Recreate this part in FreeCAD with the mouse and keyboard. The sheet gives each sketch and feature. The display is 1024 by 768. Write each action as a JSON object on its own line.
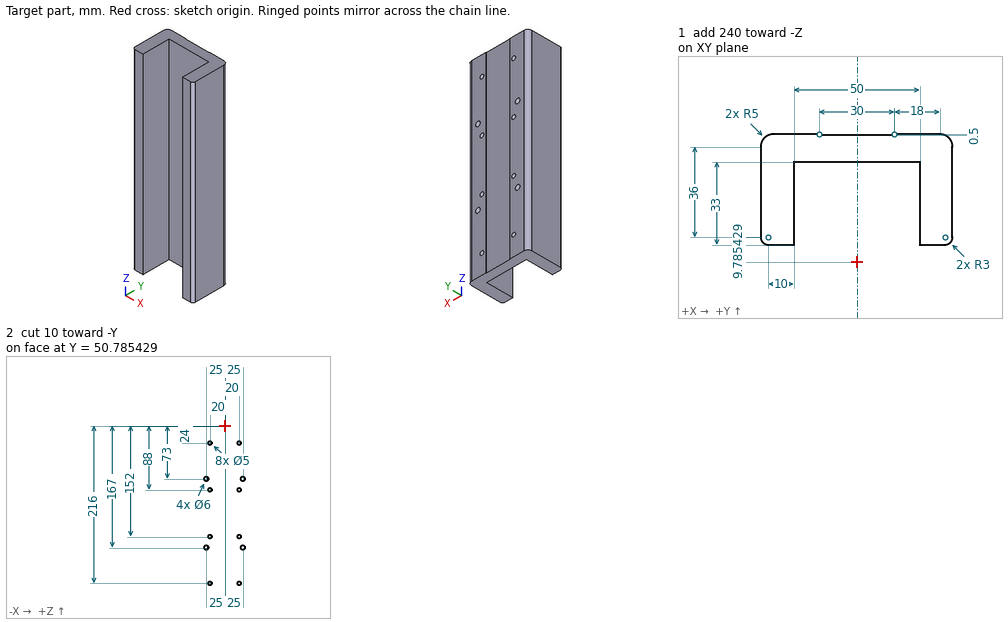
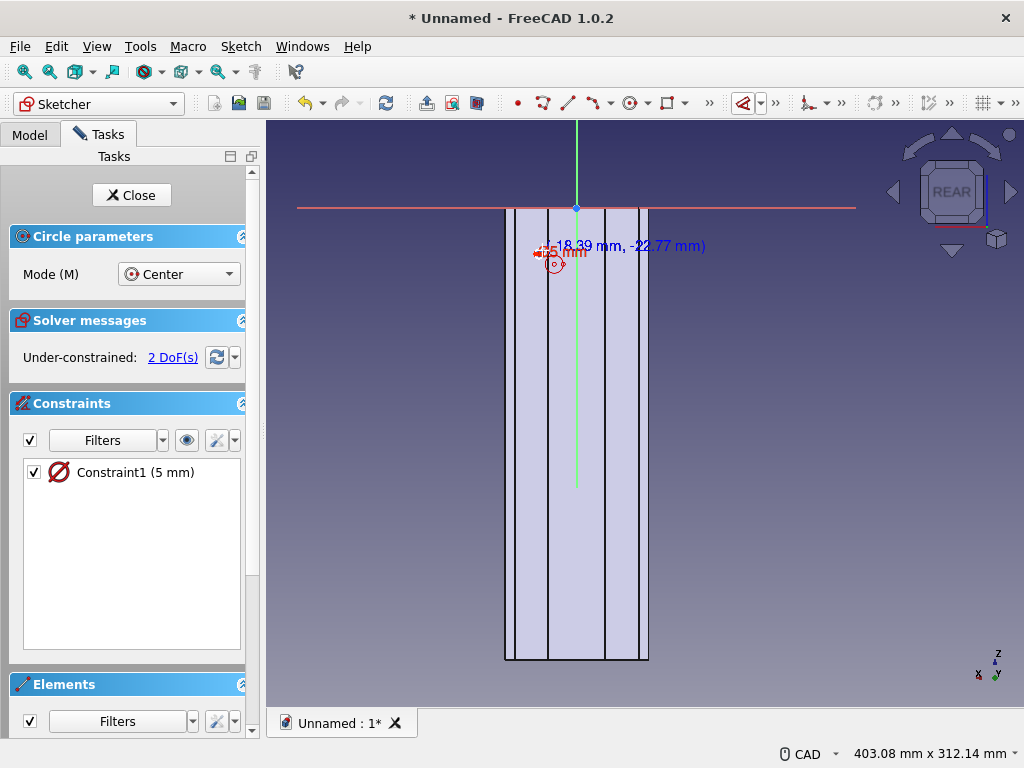
{"action": "scroll", "coordinate": [614, 253], "scroll_direction": "up", "scroll_amount": 8}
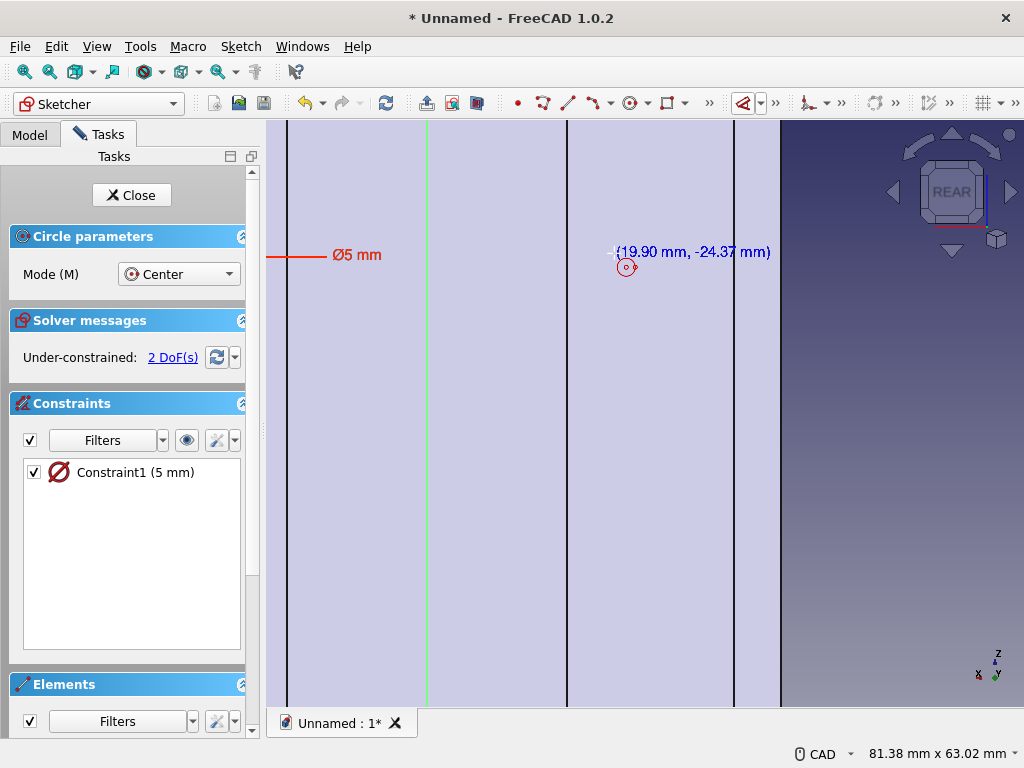
{"action": "scroll", "coordinate": [614, 253], "scroll_direction": "down", "scroll_amount": 8}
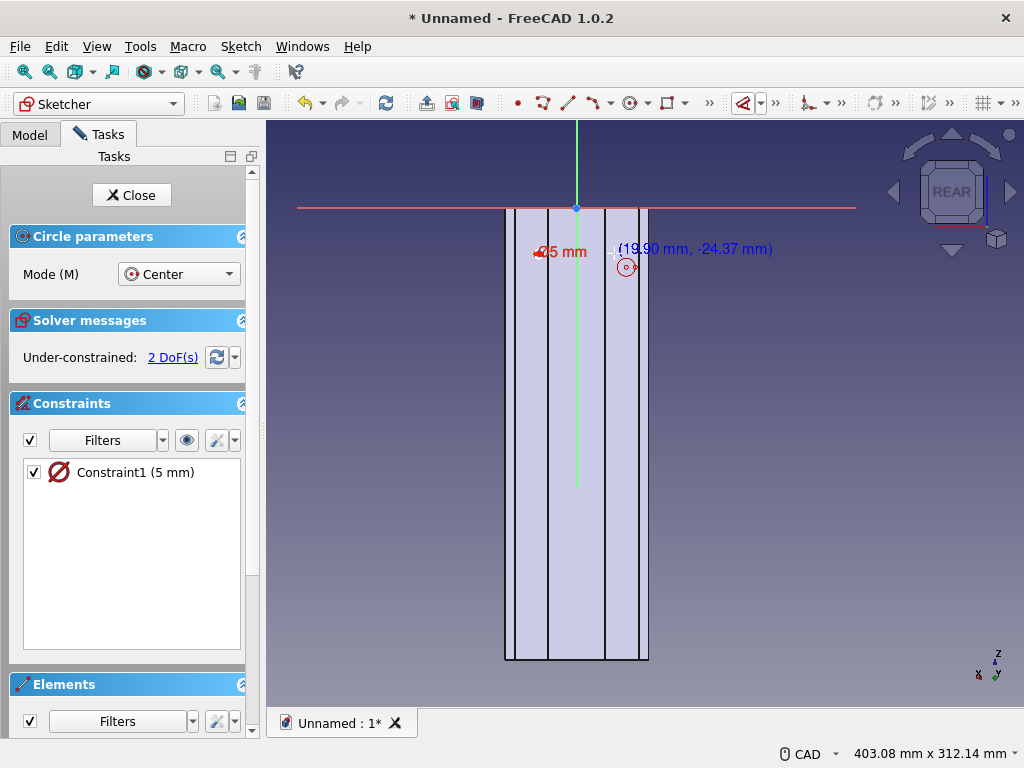
{"action": "left_click", "coordinate": [614, 253]}
{"action": "mouse_move", "coordinate": [618, 250]}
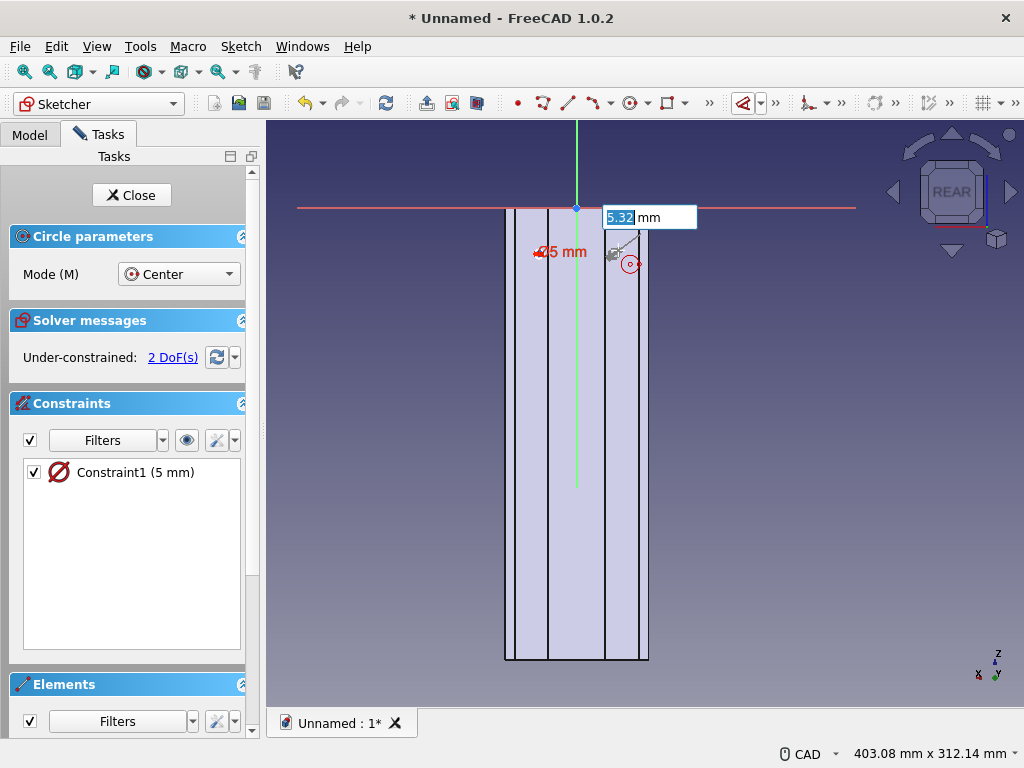
{"action": "type", "text": "5"}
{"action": "key", "text": "Return"}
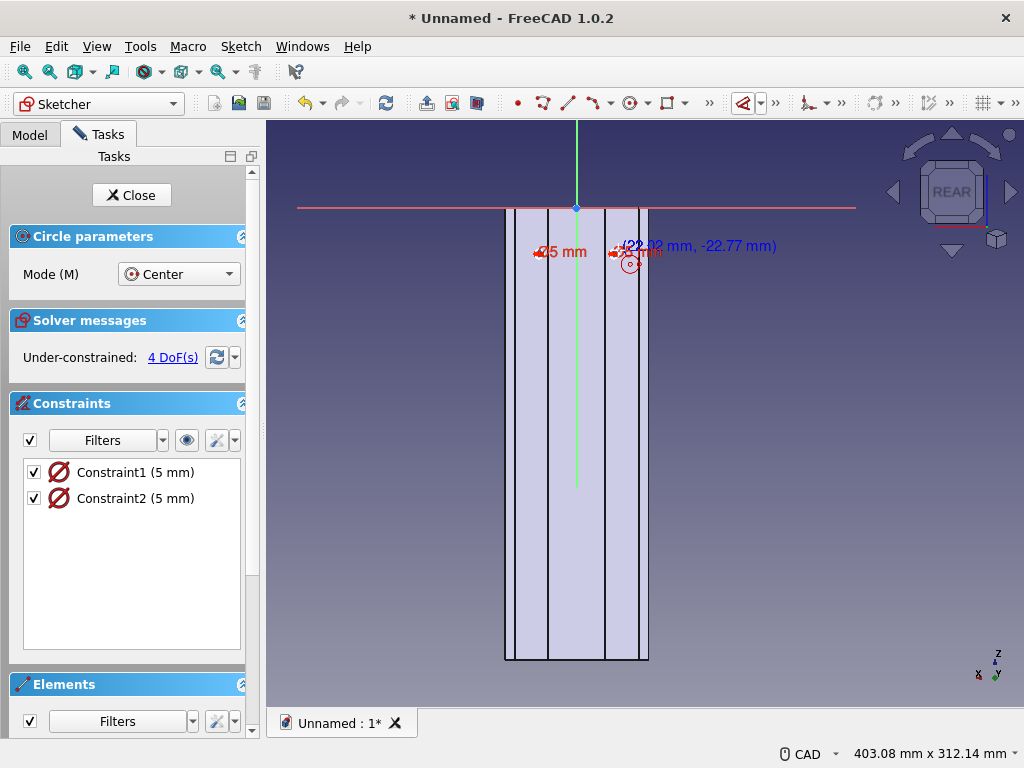
{"action": "scroll", "coordinate": [539, 374], "scroll_direction": "up", "scroll_amount": 8}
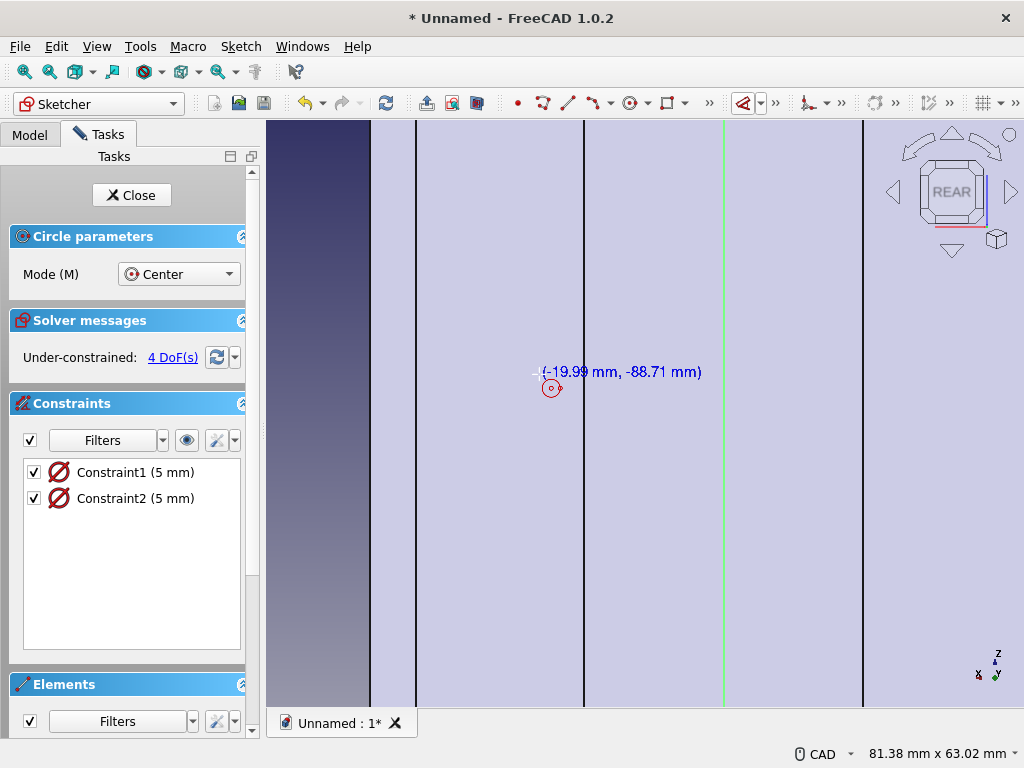
{"action": "scroll", "coordinate": [539, 374], "scroll_direction": "down", "scroll_amount": 8}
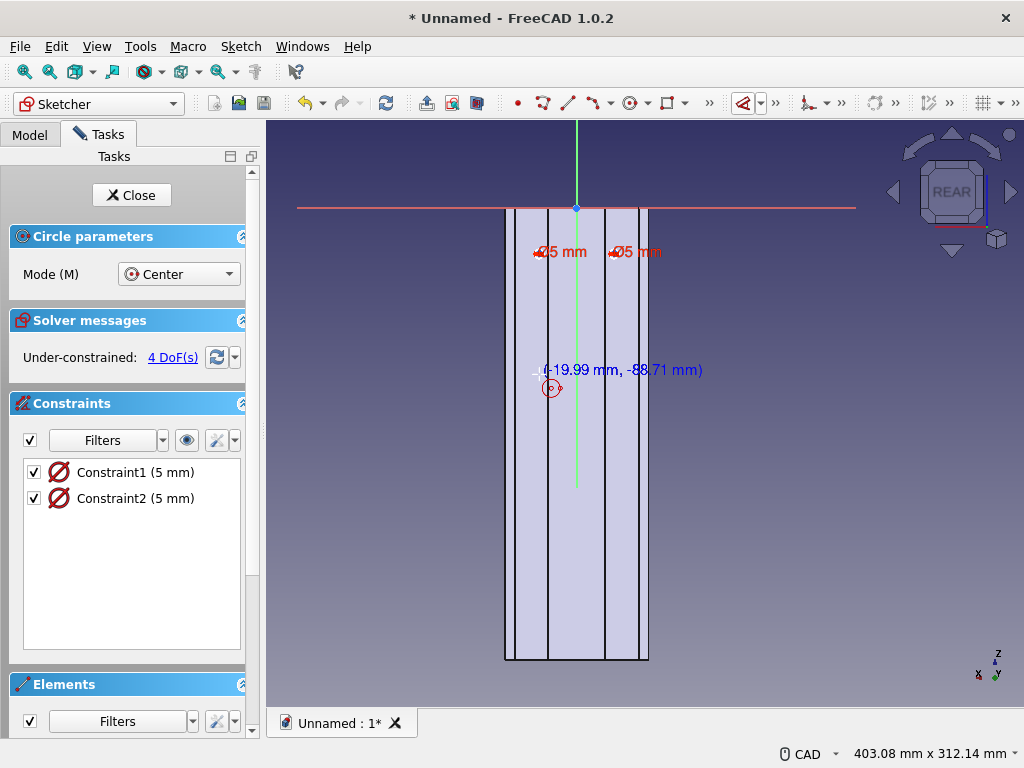
{"action": "left_click", "coordinate": [539, 374]}
{"action": "mouse_move", "coordinate": [542, 370]}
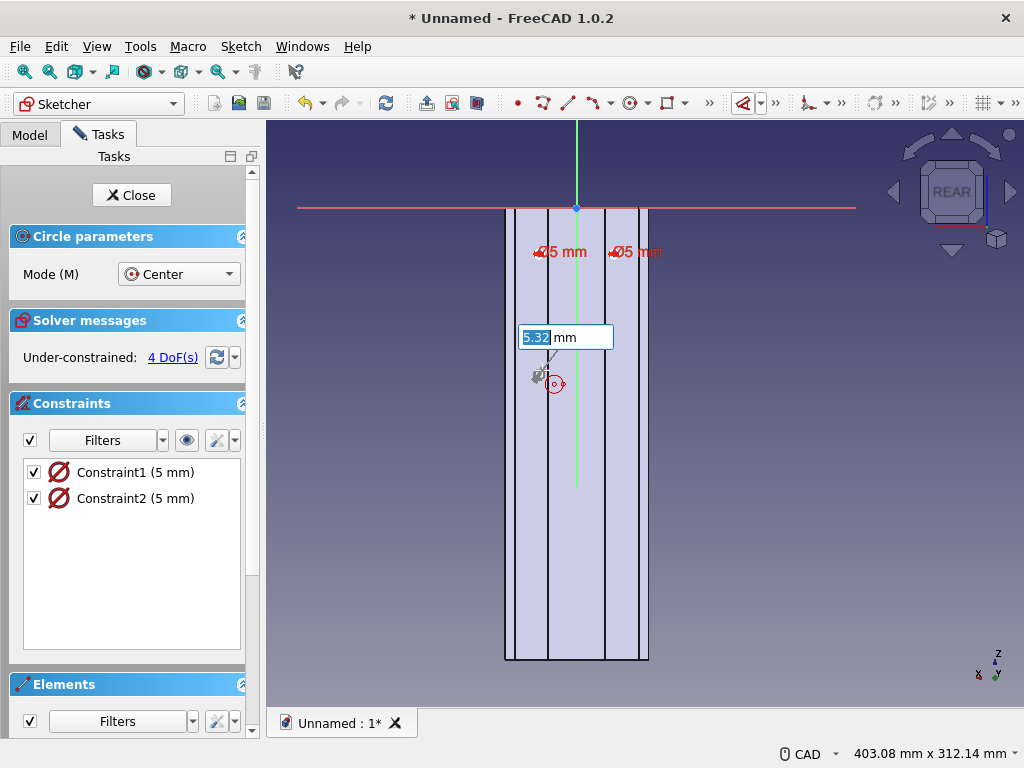
{"action": "type", "text": "5"}
{"action": "key", "text": "Return"}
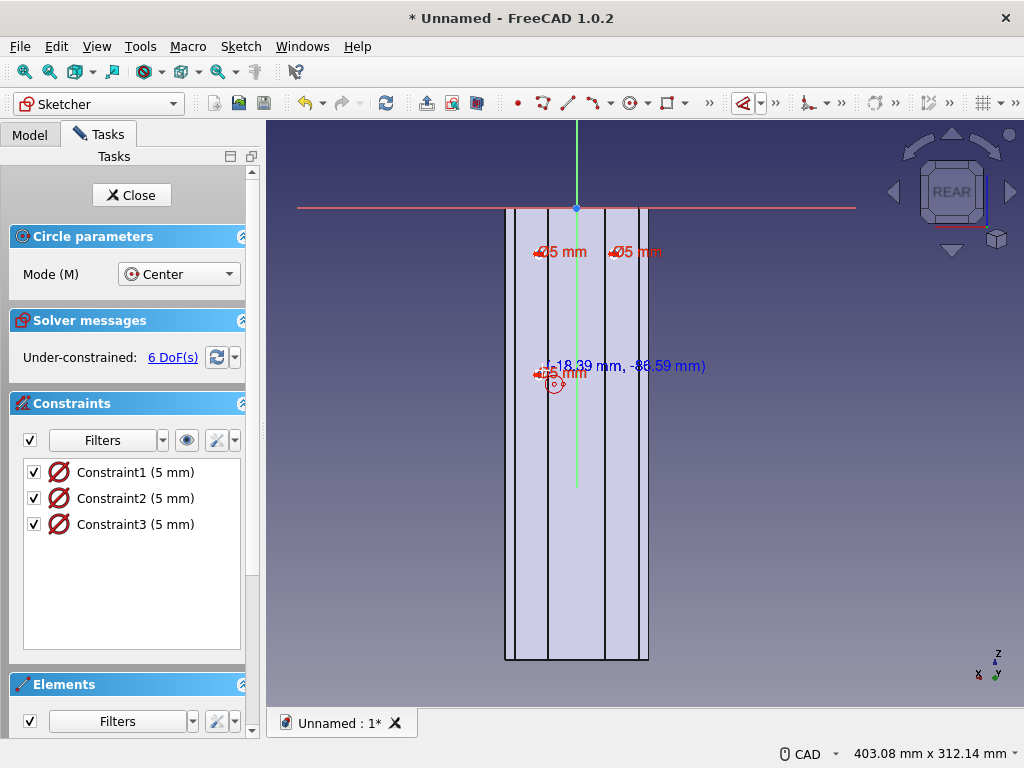
{"action": "scroll", "coordinate": [614, 374], "scroll_direction": "up", "scroll_amount": 8}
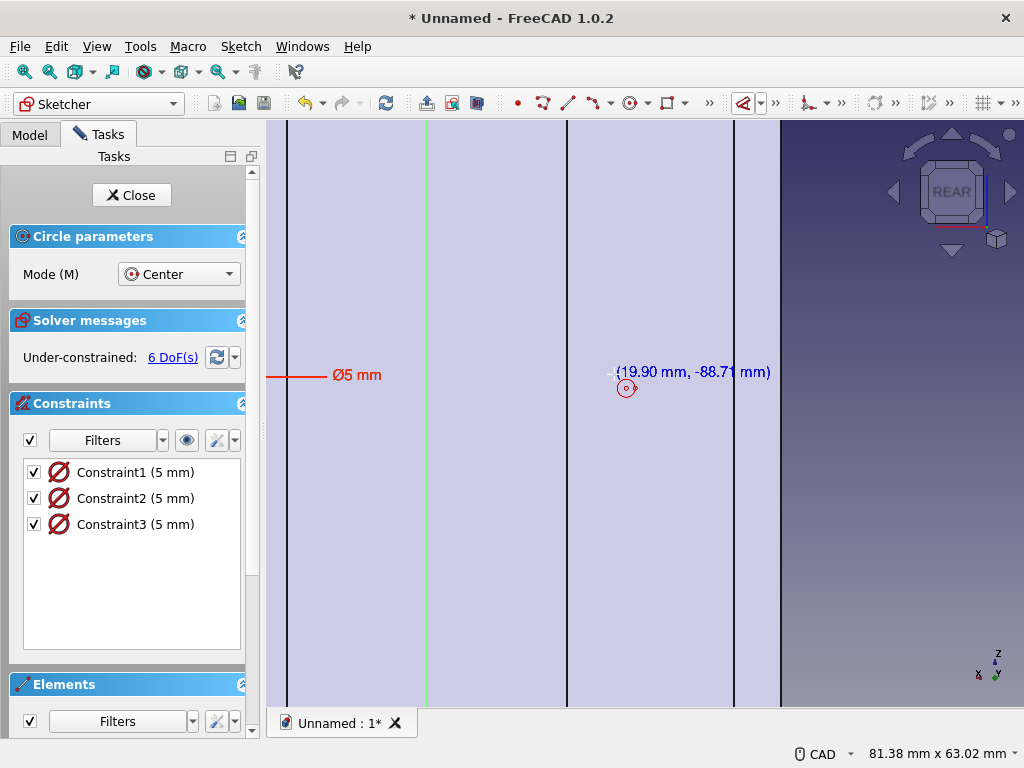
{"action": "scroll", "coordinate": [614, 374], "scroll_direction": "down", "scroll_amount": 8}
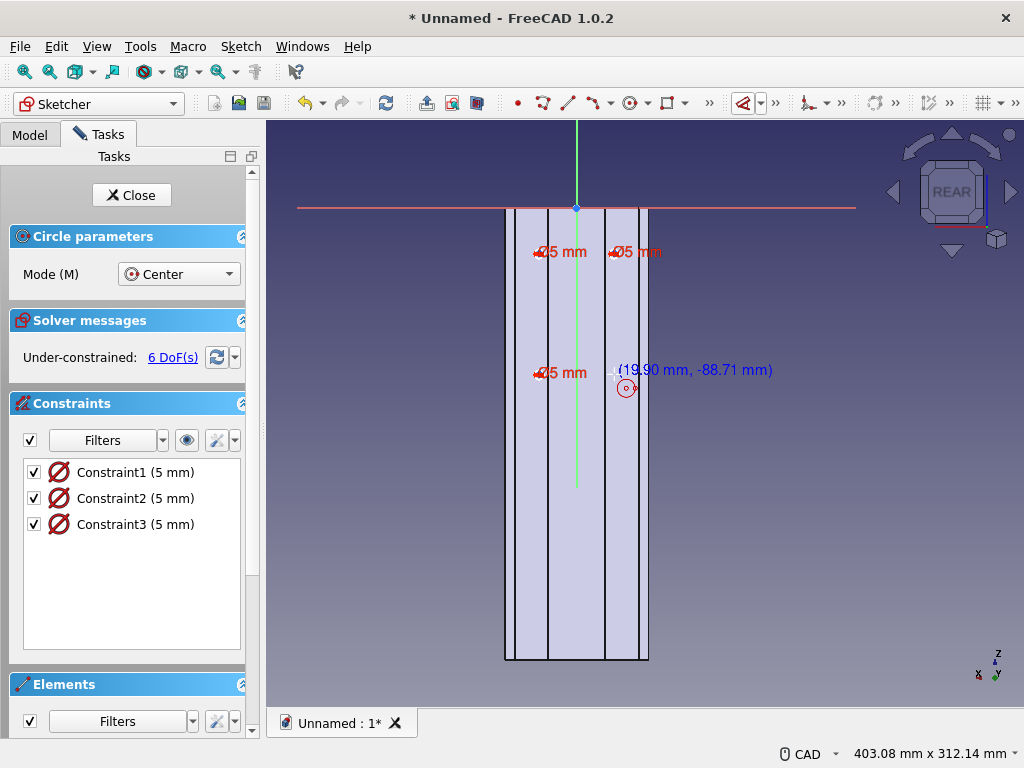
{"action": "left_click", "coordinate": [614, 374]}
{"action": "mouse_move", "coordinate": [618, 370]}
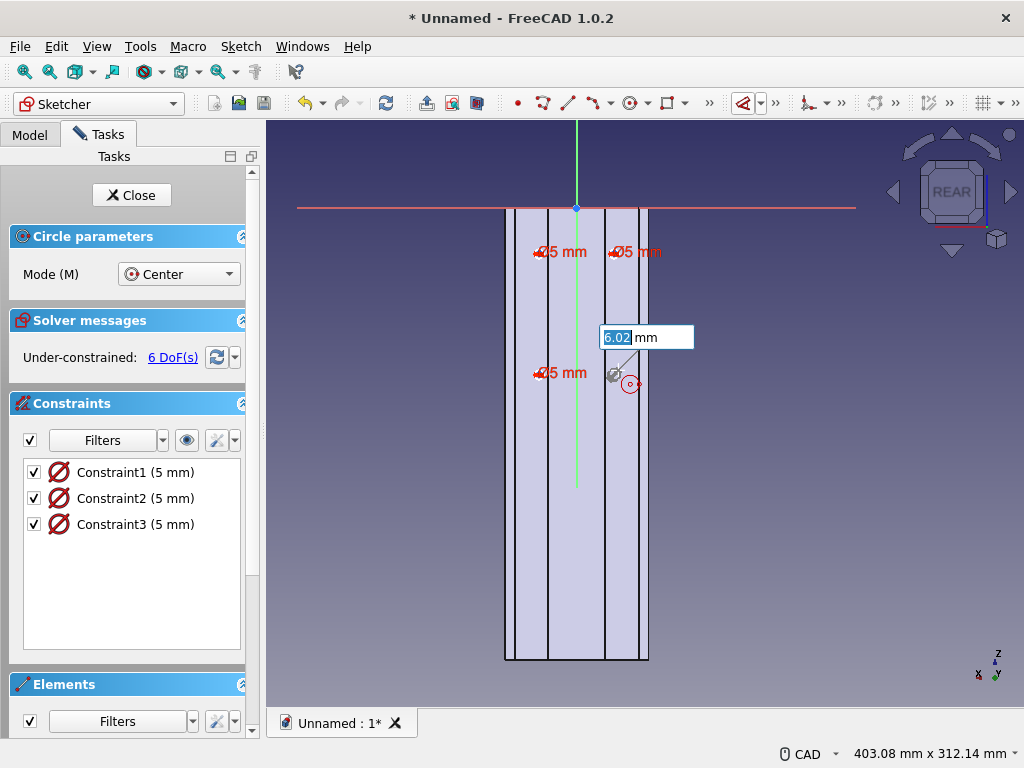
{"action": "type", "text": "5"}
{"action": "key", "text": "Return"}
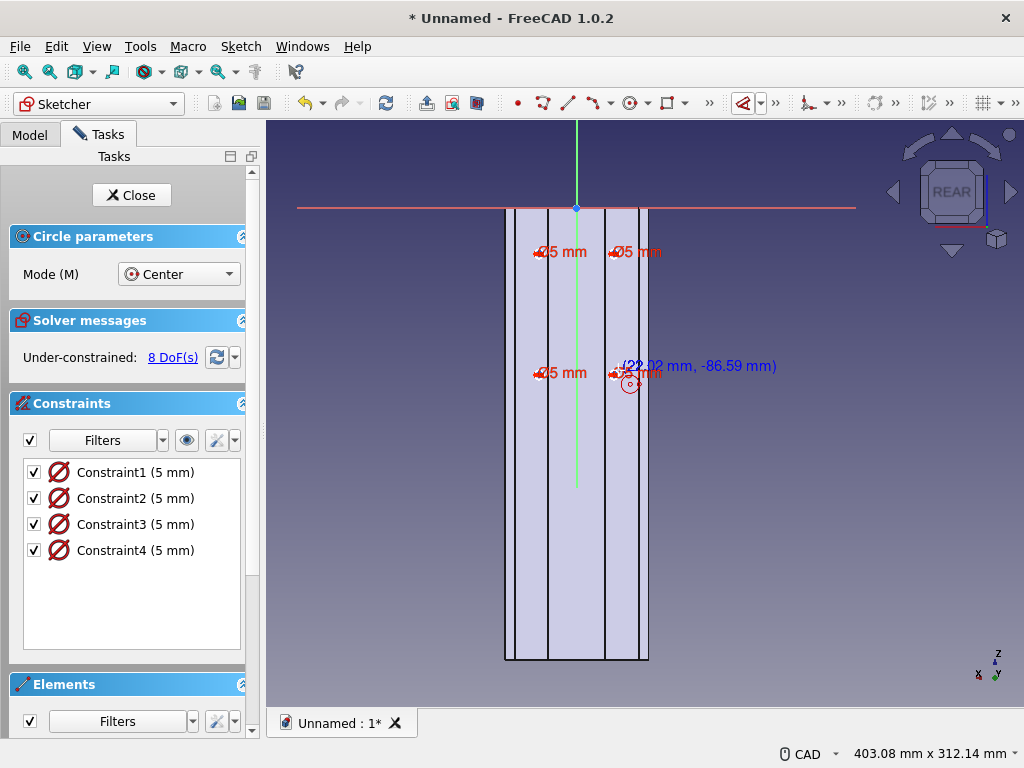
{"action": "scroll", "coordinate": [539, 494], "scroll_direction": "up", "scroll_amount": 8}